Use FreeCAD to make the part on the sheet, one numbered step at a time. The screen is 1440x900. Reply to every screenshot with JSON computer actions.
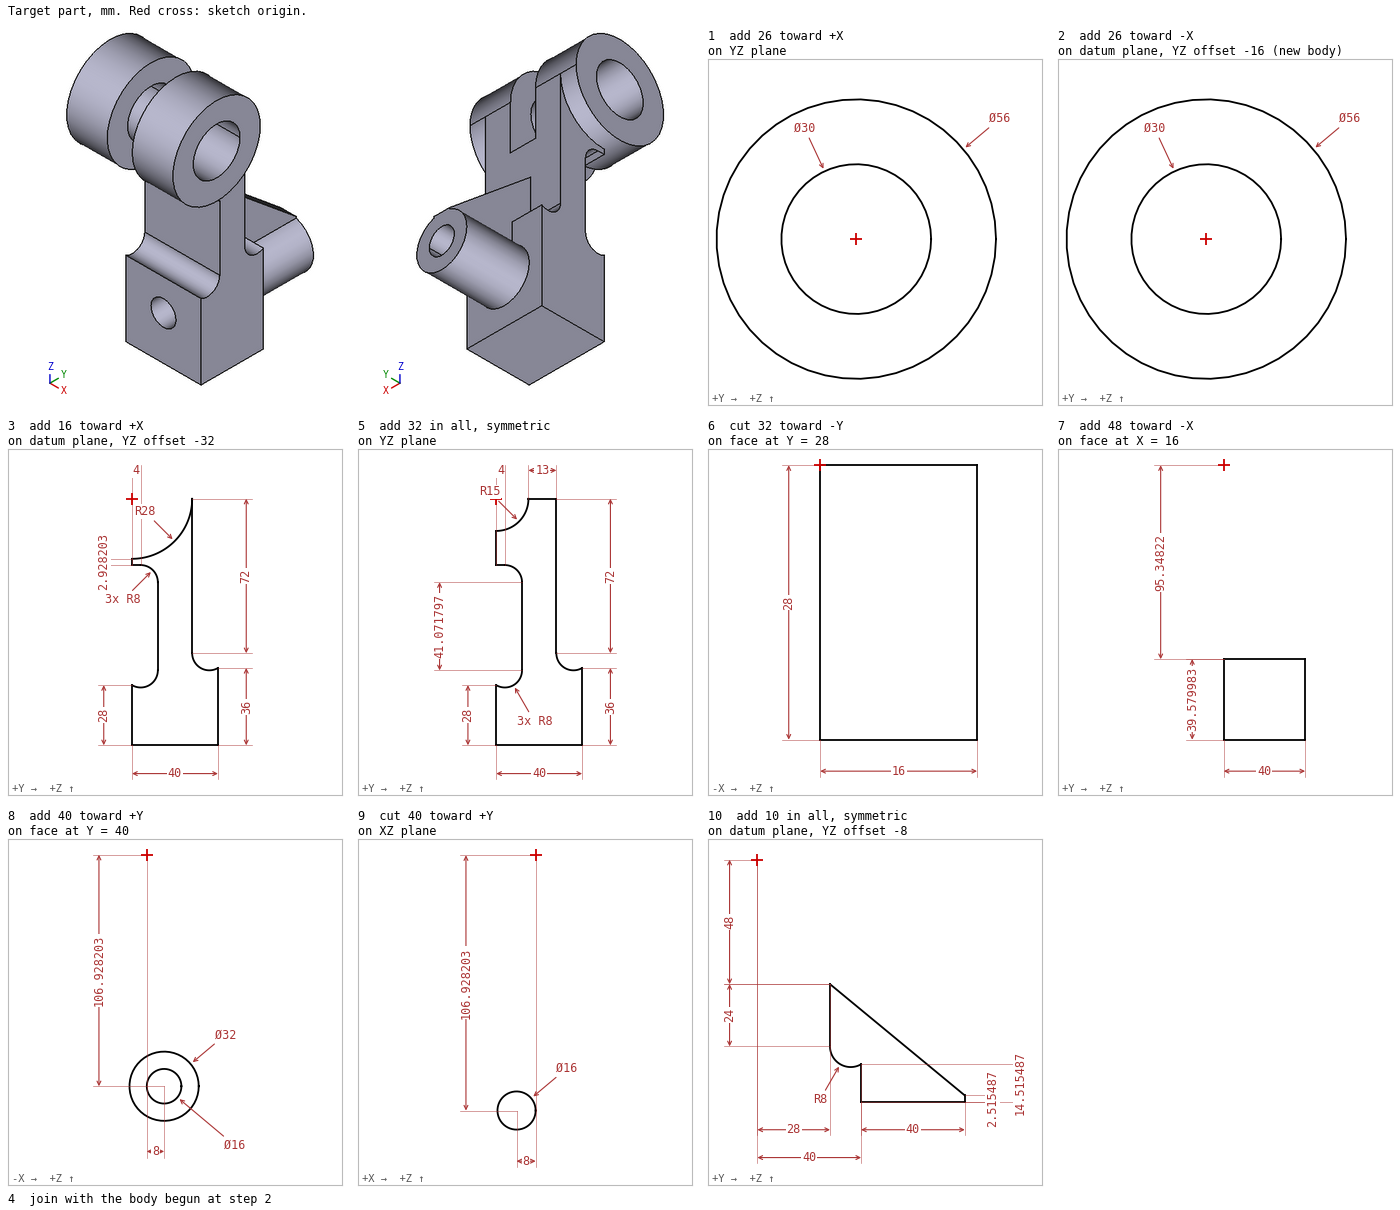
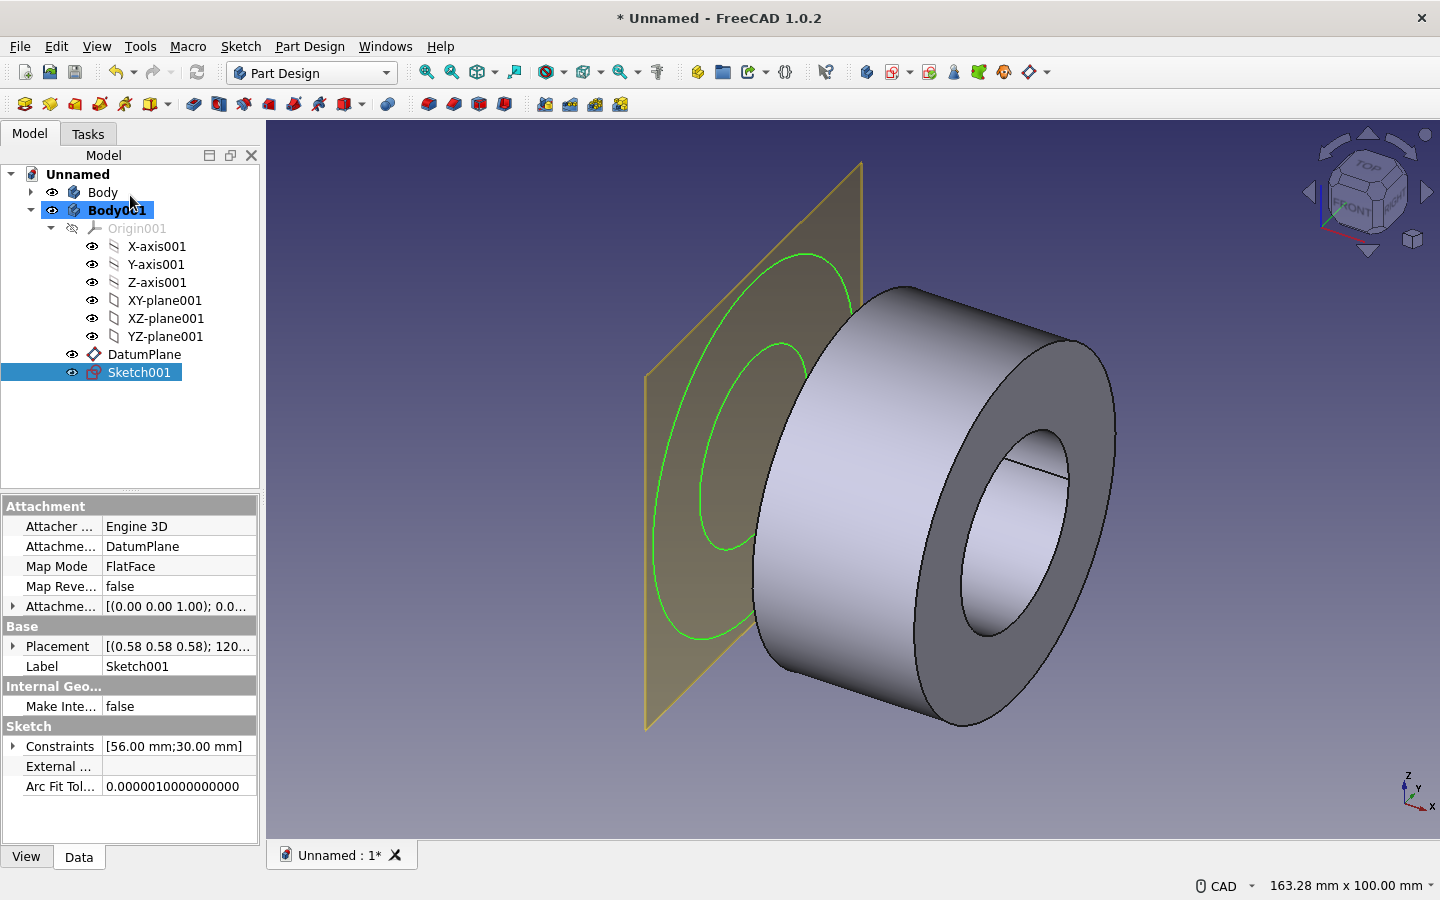
{"action": "left_click", "coordinate": [25, 104]}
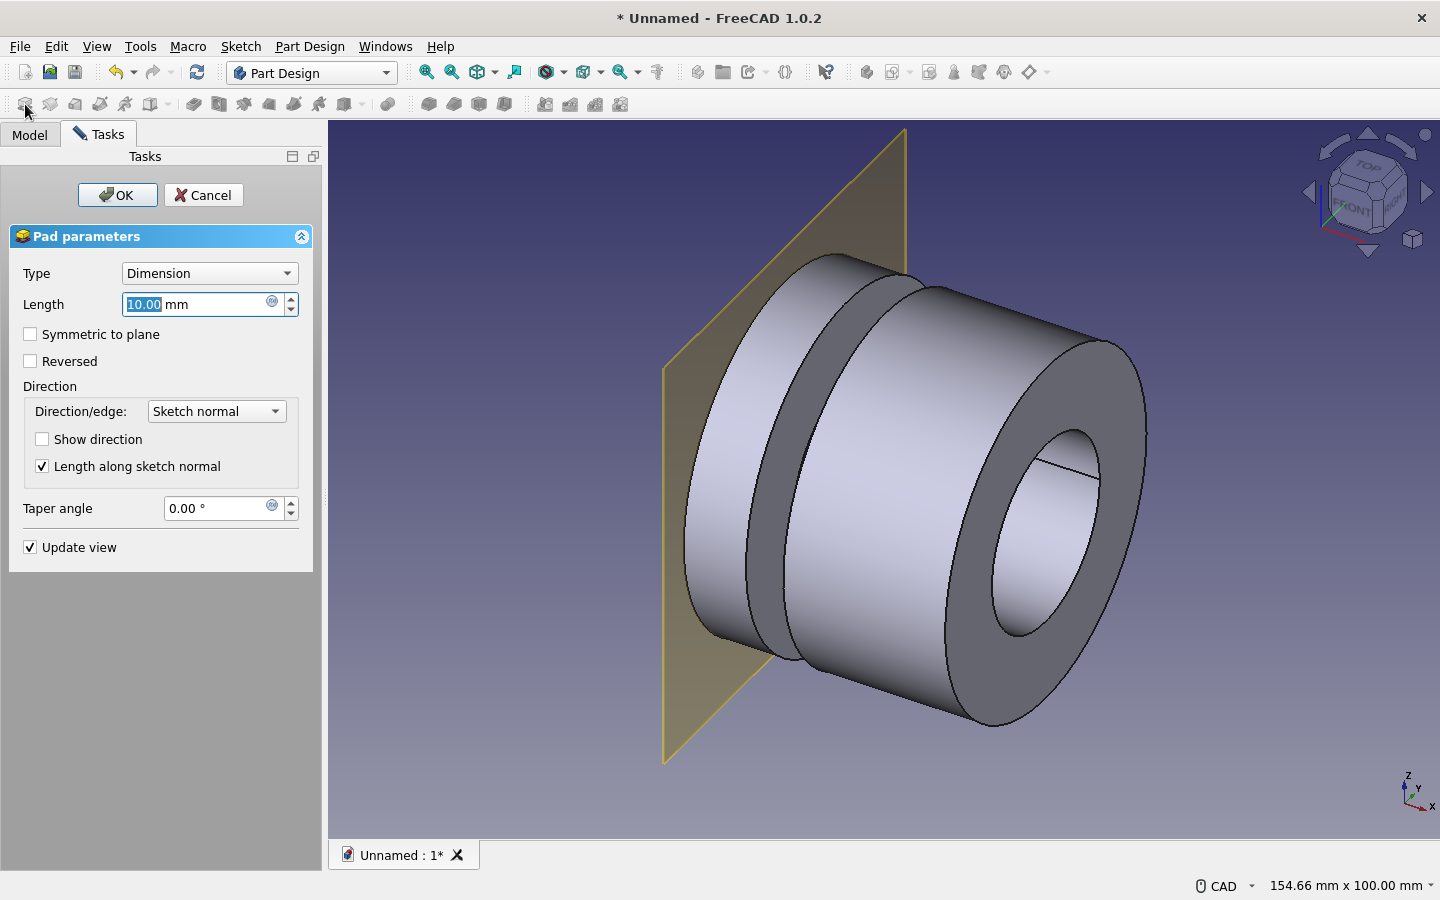
{"action": "type", "text": "26"}
{"action": "key", "text": "Tab"}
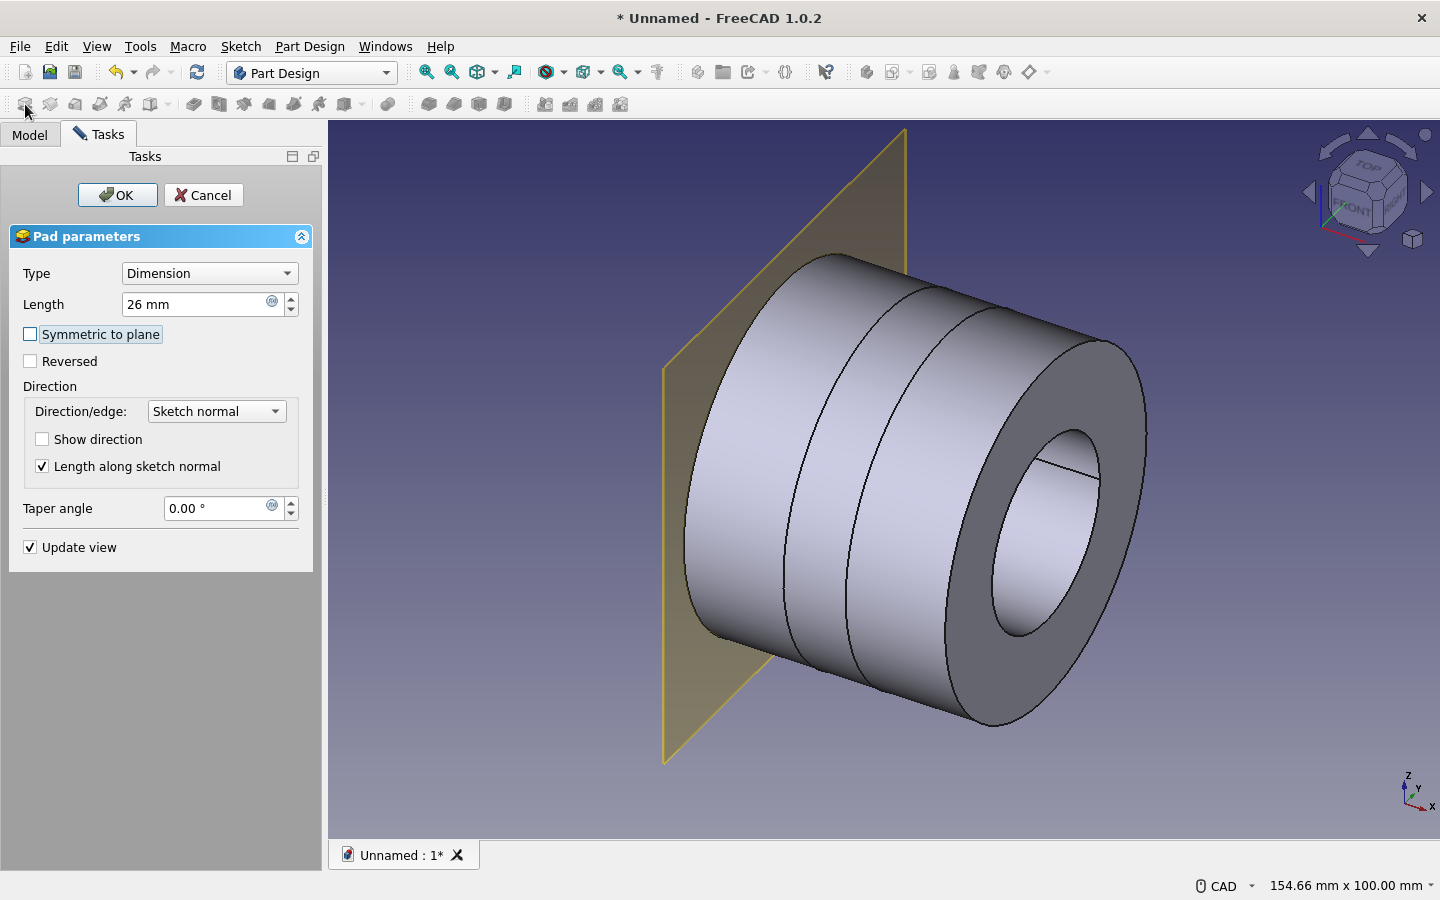
{"action": "left_click", "coordinate": [31, 361]}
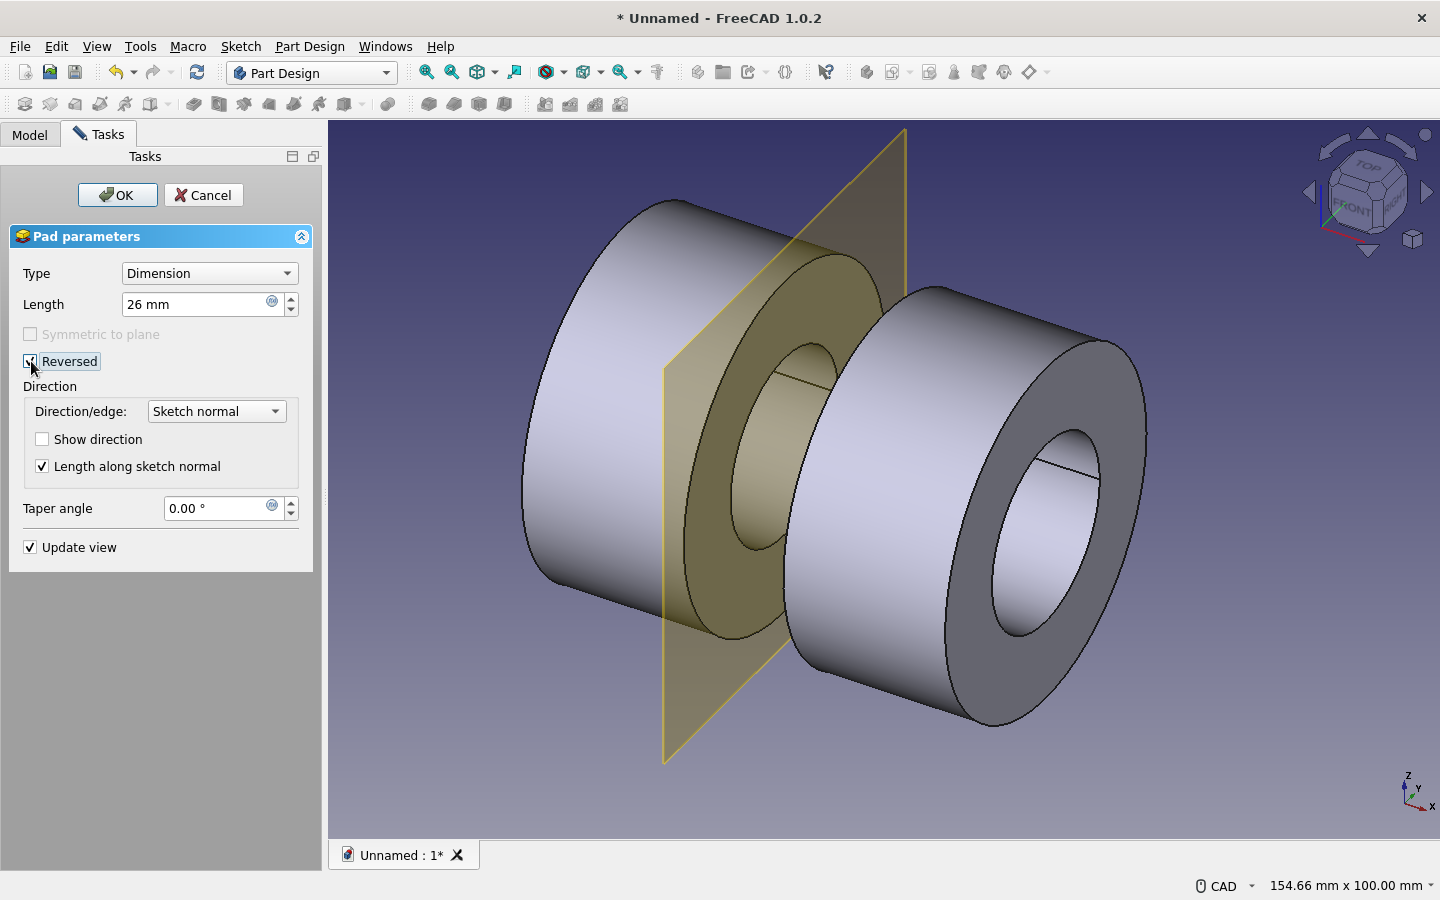
{"action": "left_click", "coordinate": [118, 195]}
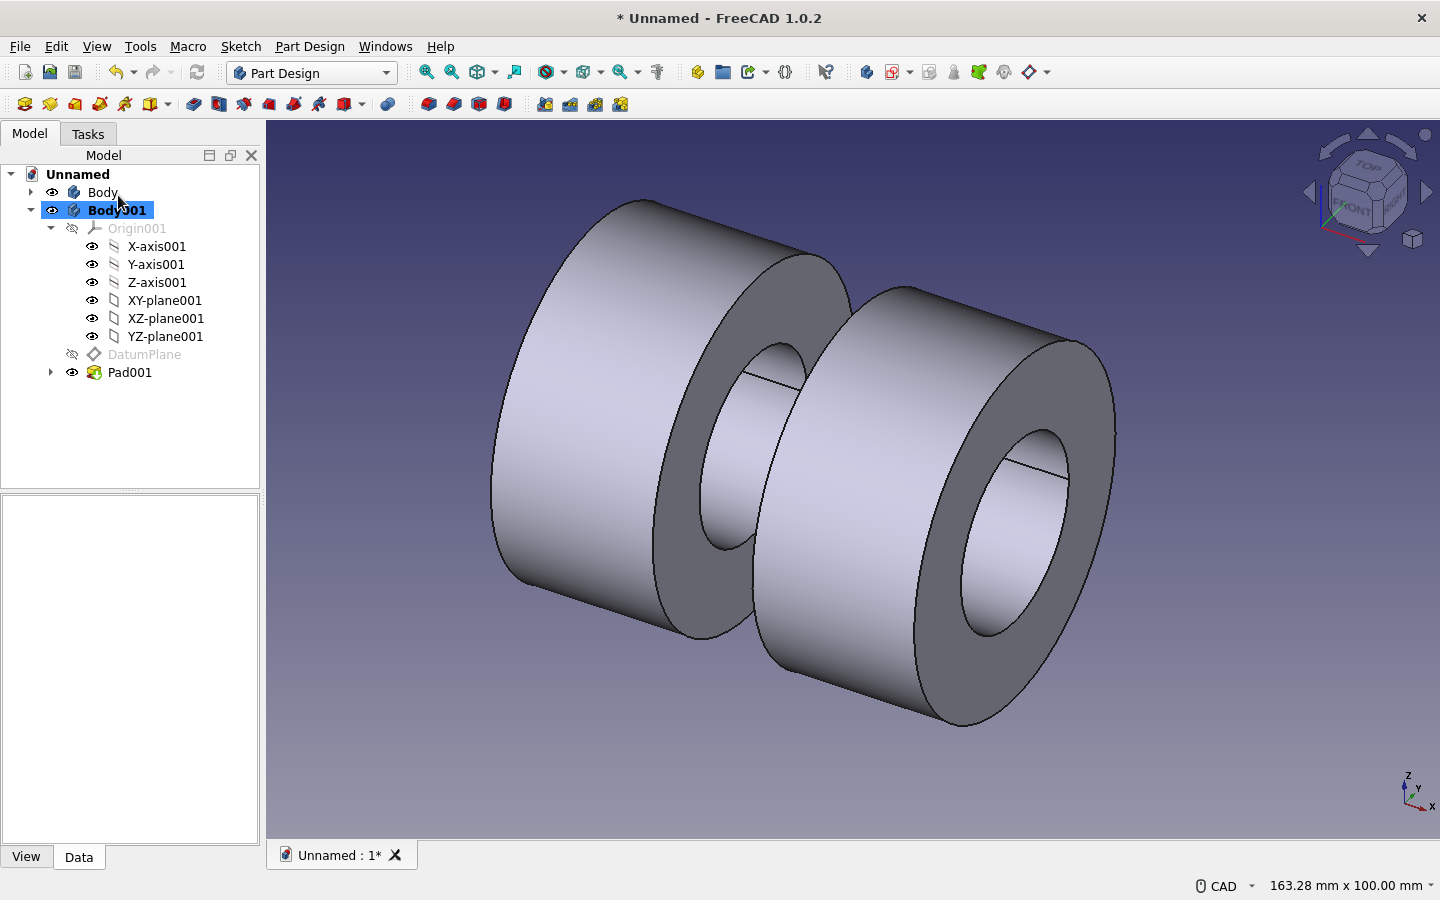
{"action": "left_click", "coordinate": [137, 336]}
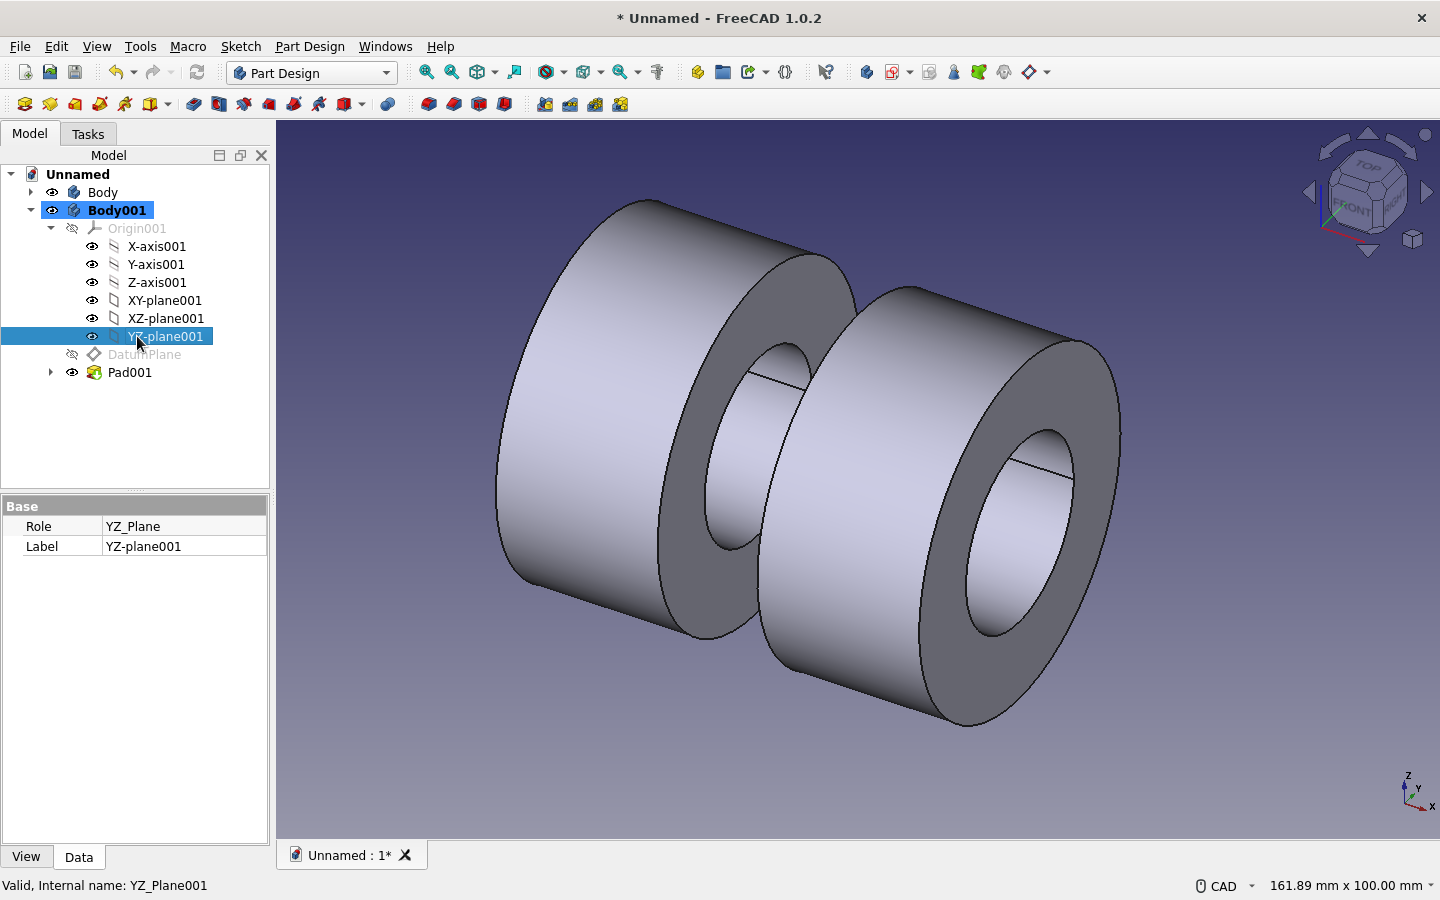
{"action": "left_click", "coordinate": [1028, 72]}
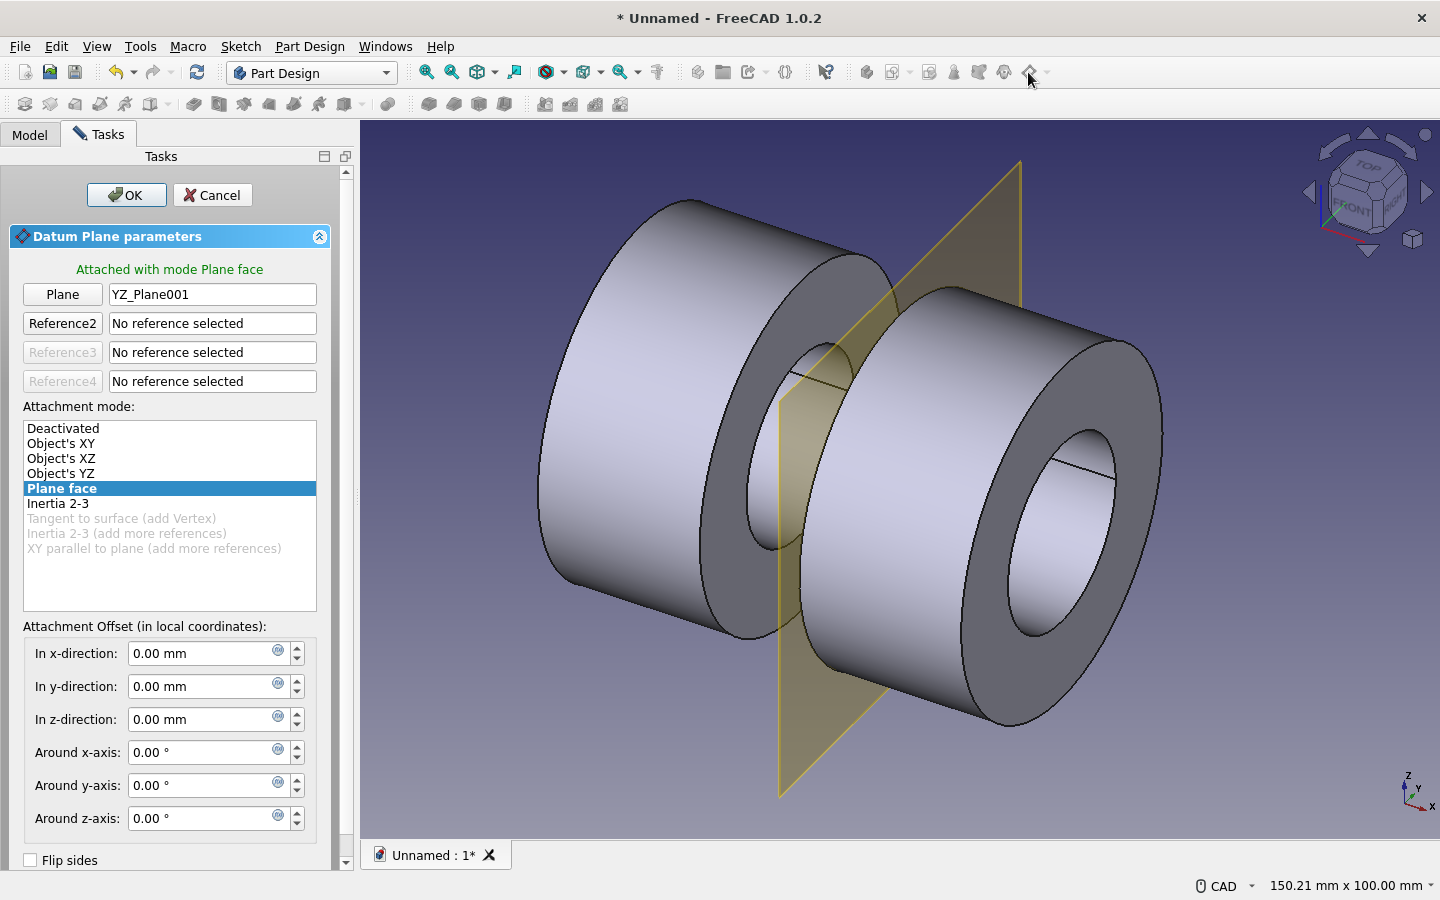
{"action": "triple_click", "coordinate": [210, 720]}